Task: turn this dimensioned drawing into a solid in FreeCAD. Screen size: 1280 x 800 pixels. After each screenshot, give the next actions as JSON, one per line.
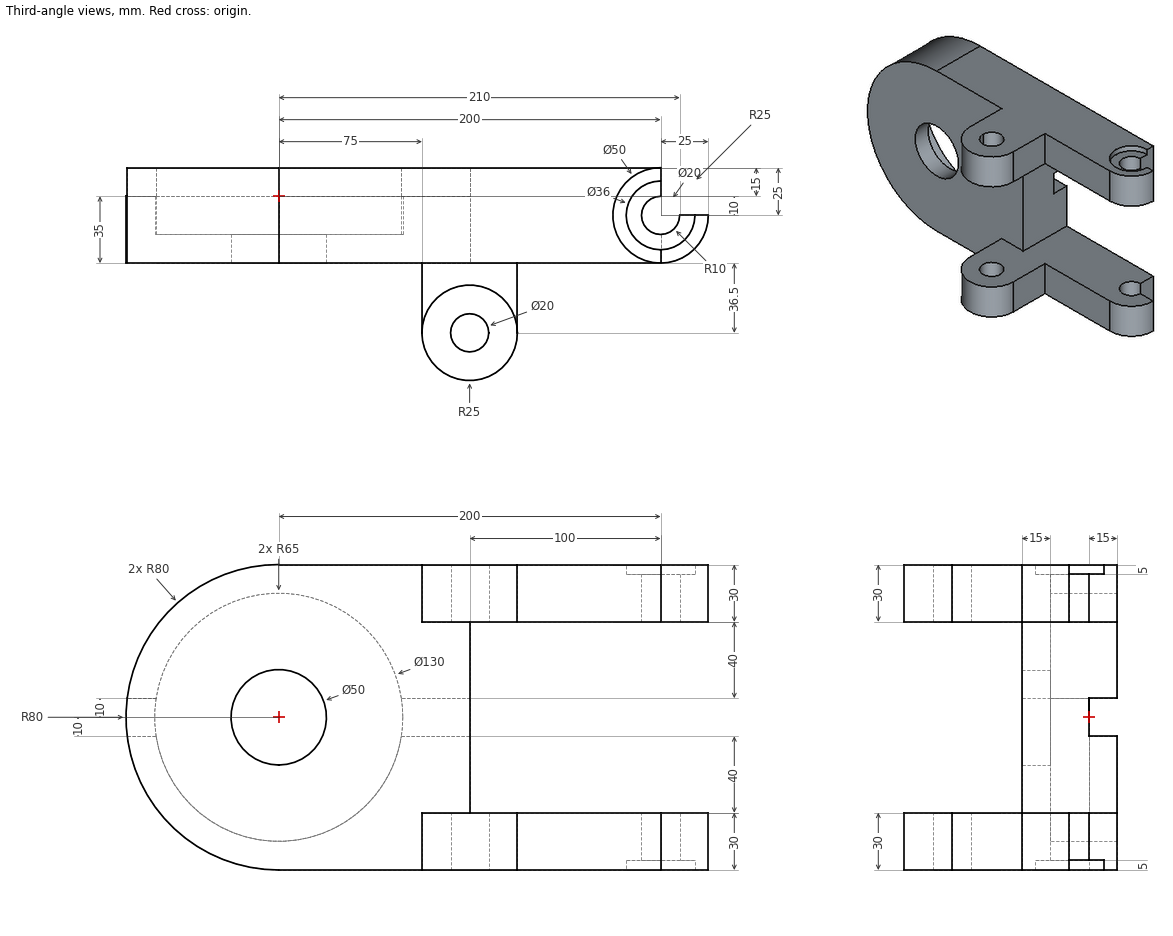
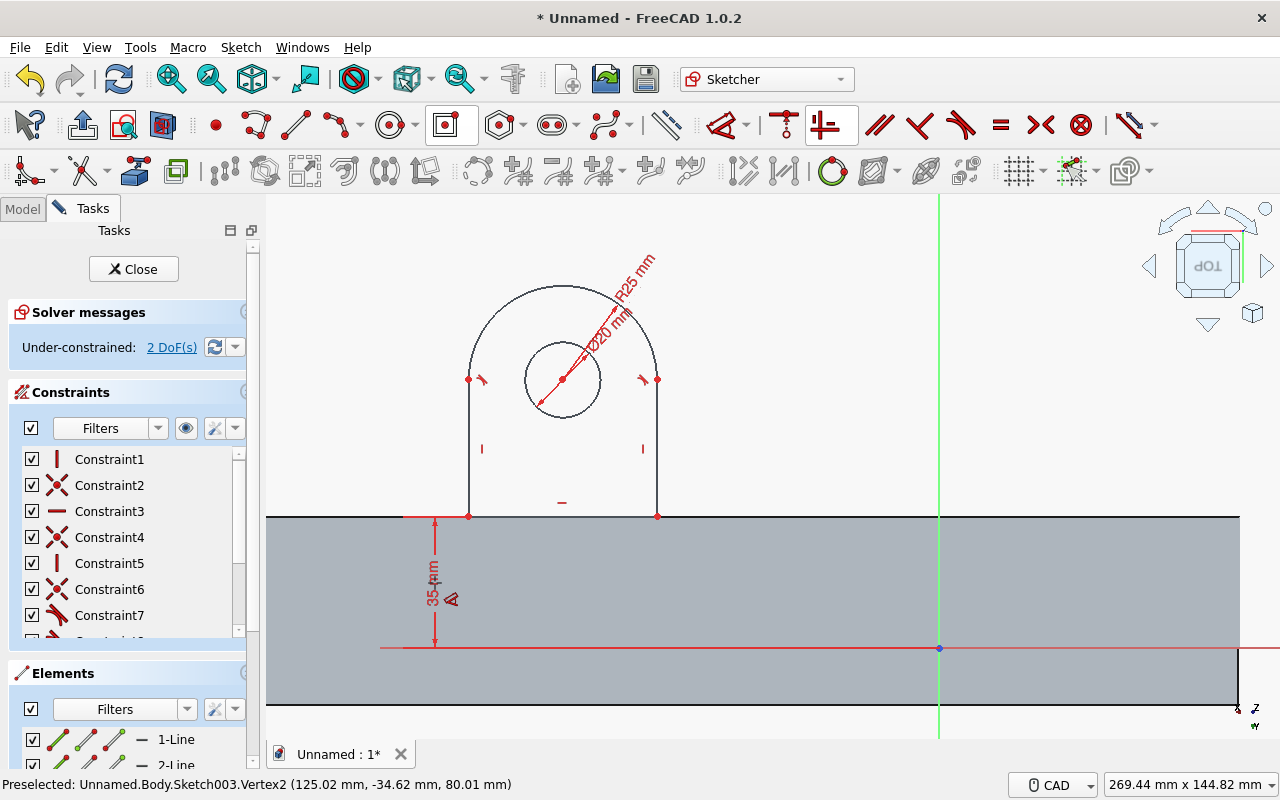
{"action": "left_click", "coordinate": [657, 517]}
{"action": "left_click", "coordinate": [798, 682]}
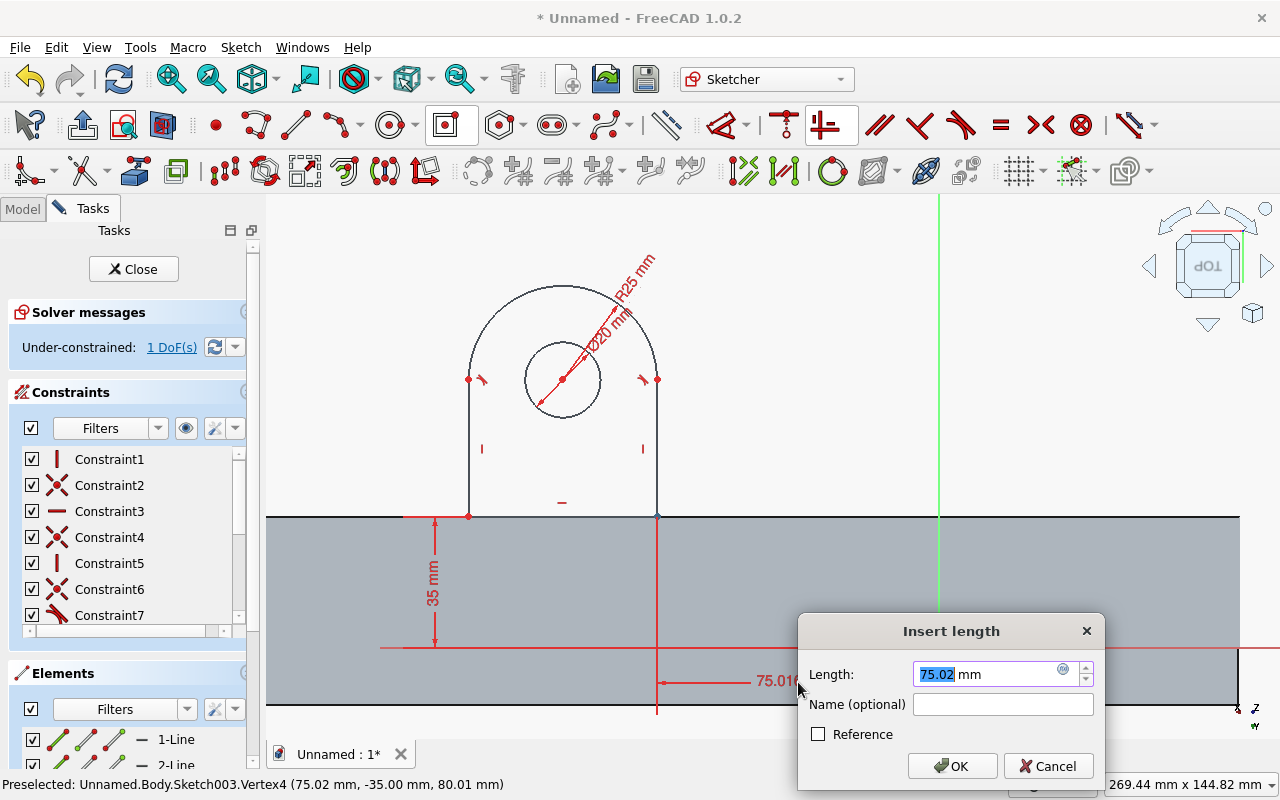
{"action": "type", "text": "75"}
{"action": "key", "text": "Return"}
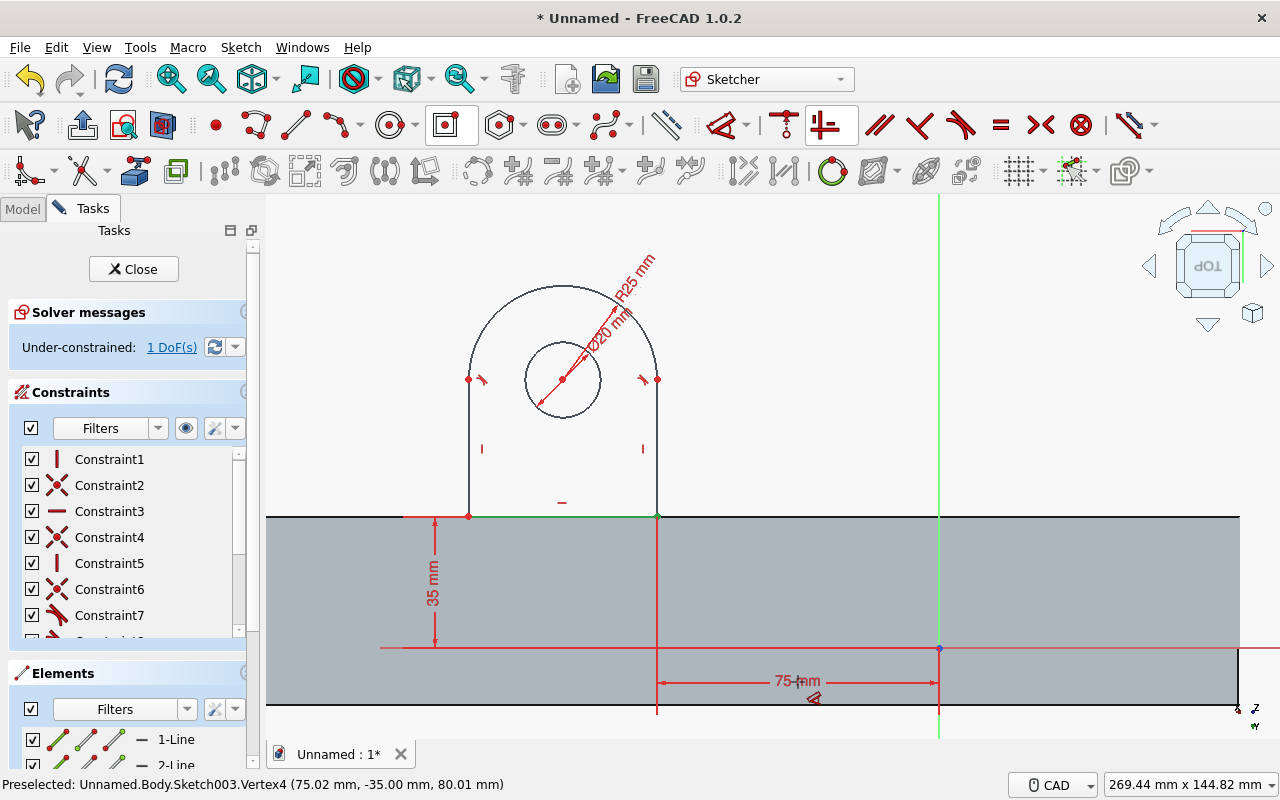
{"action": "left_click", "coordinate": [469, 421]}
{"action": "left_click", "coordinate": [435, 448]}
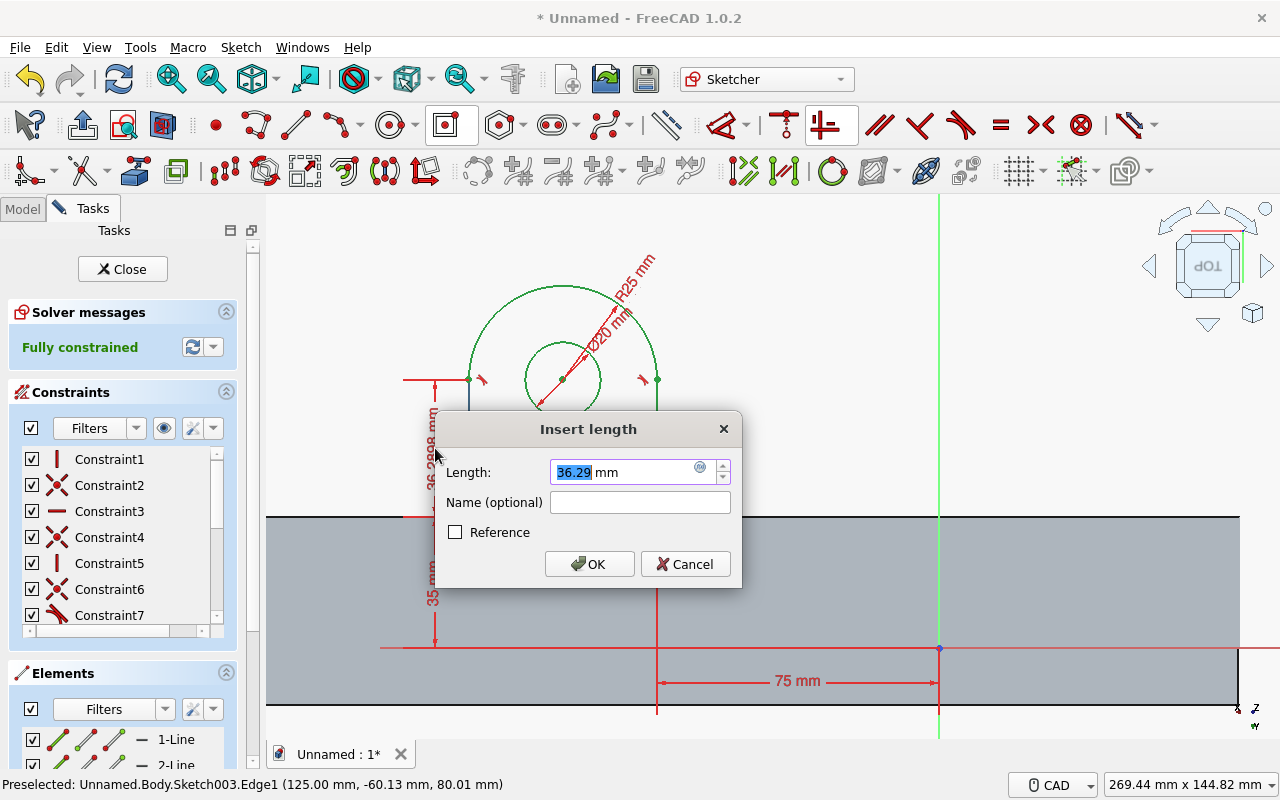
{"action": "type", "text": "36.5"}
{"action": "key", "text": "Return"}
{"action": "key", "text": "Escape"}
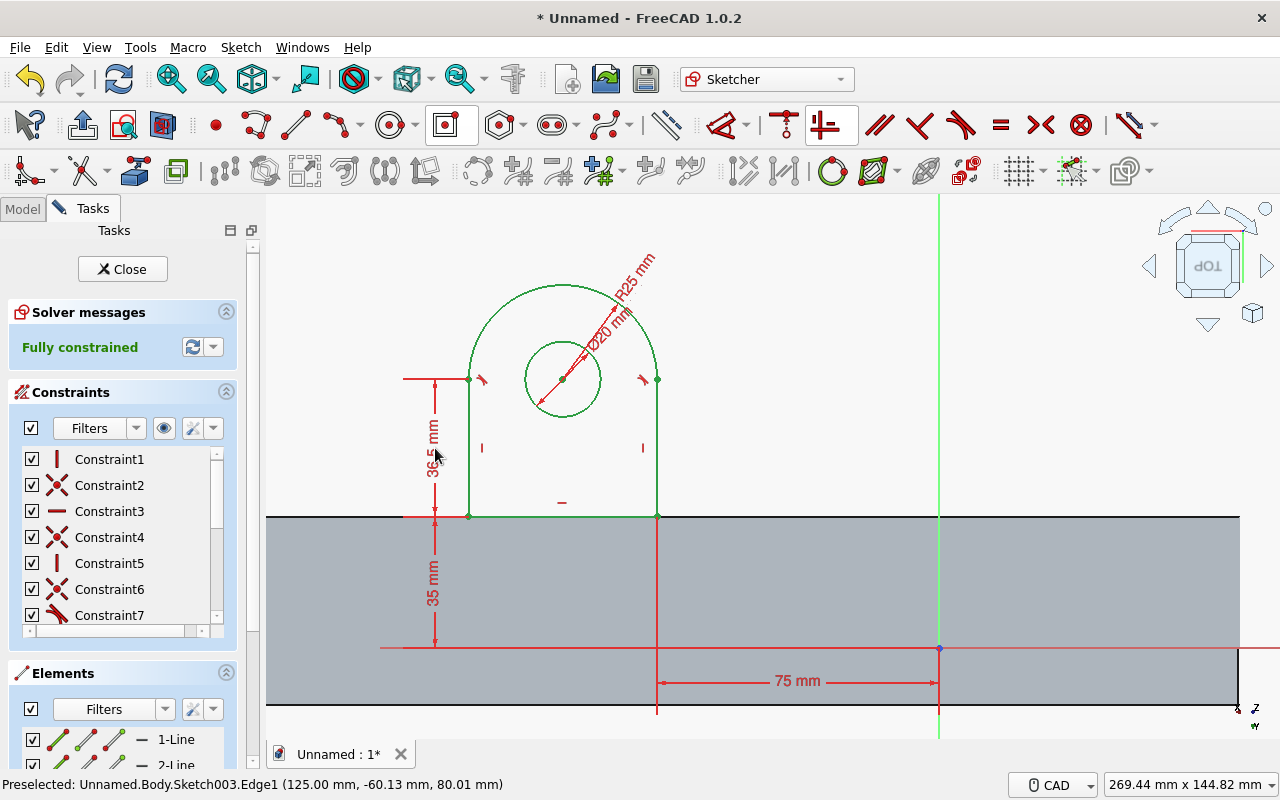
{"action": "left_click", "coordinate": [123, 269]}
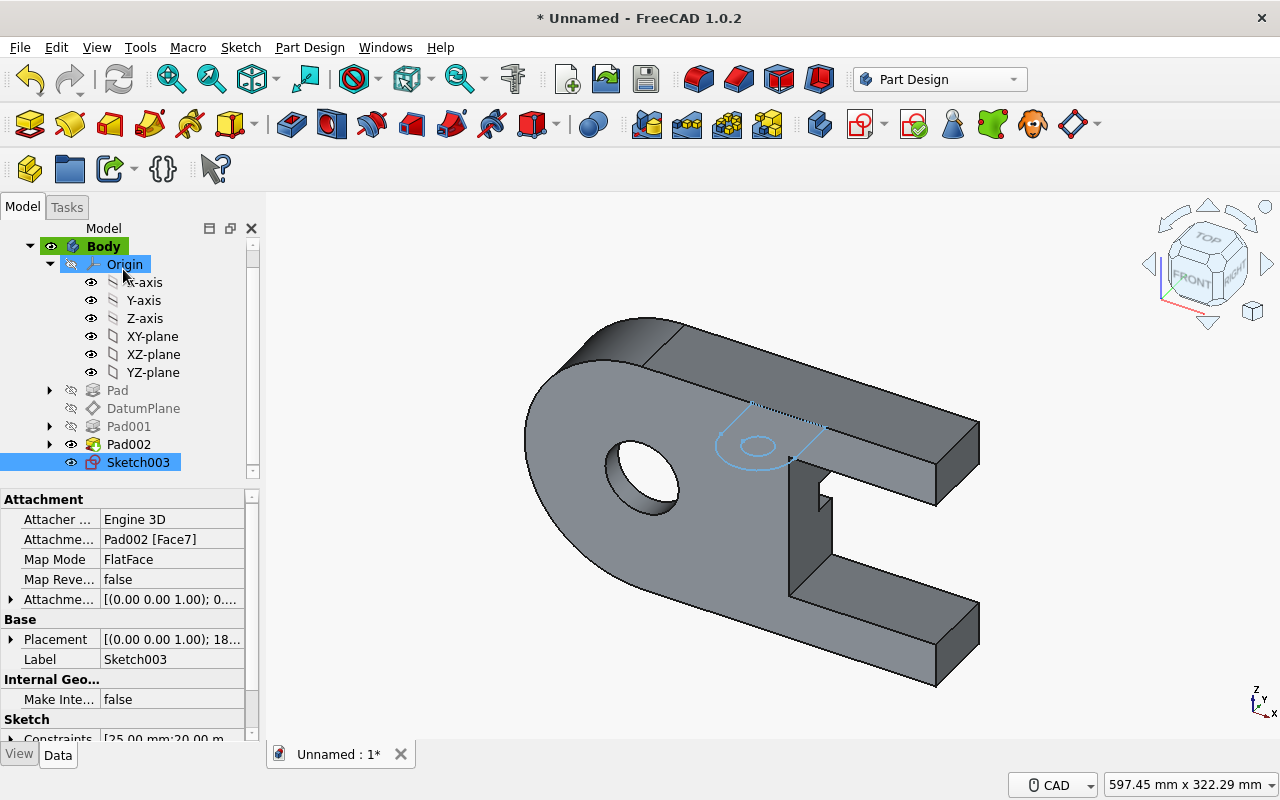
{"action": "left_click", "coordinate": [30, 124]}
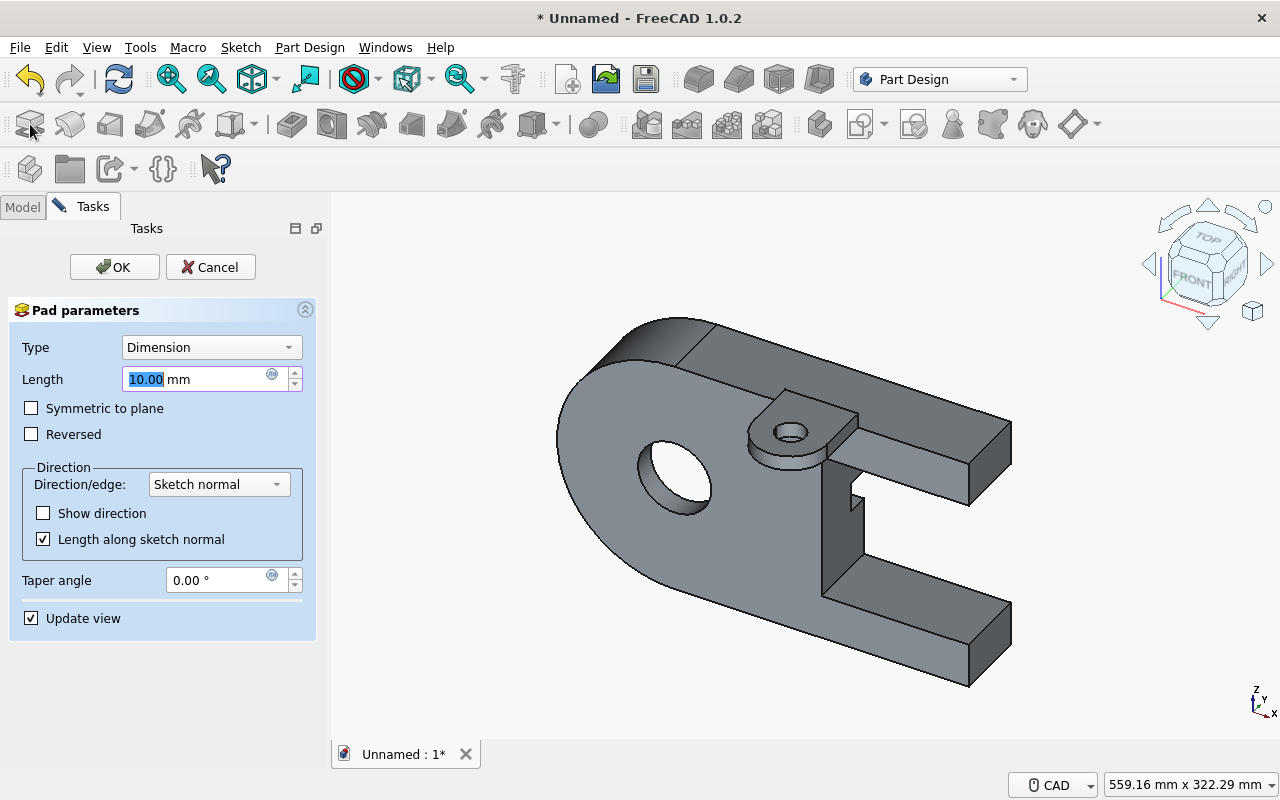
{"action": "type", "text": "30"}
{"action": "key", "text": "Tab"}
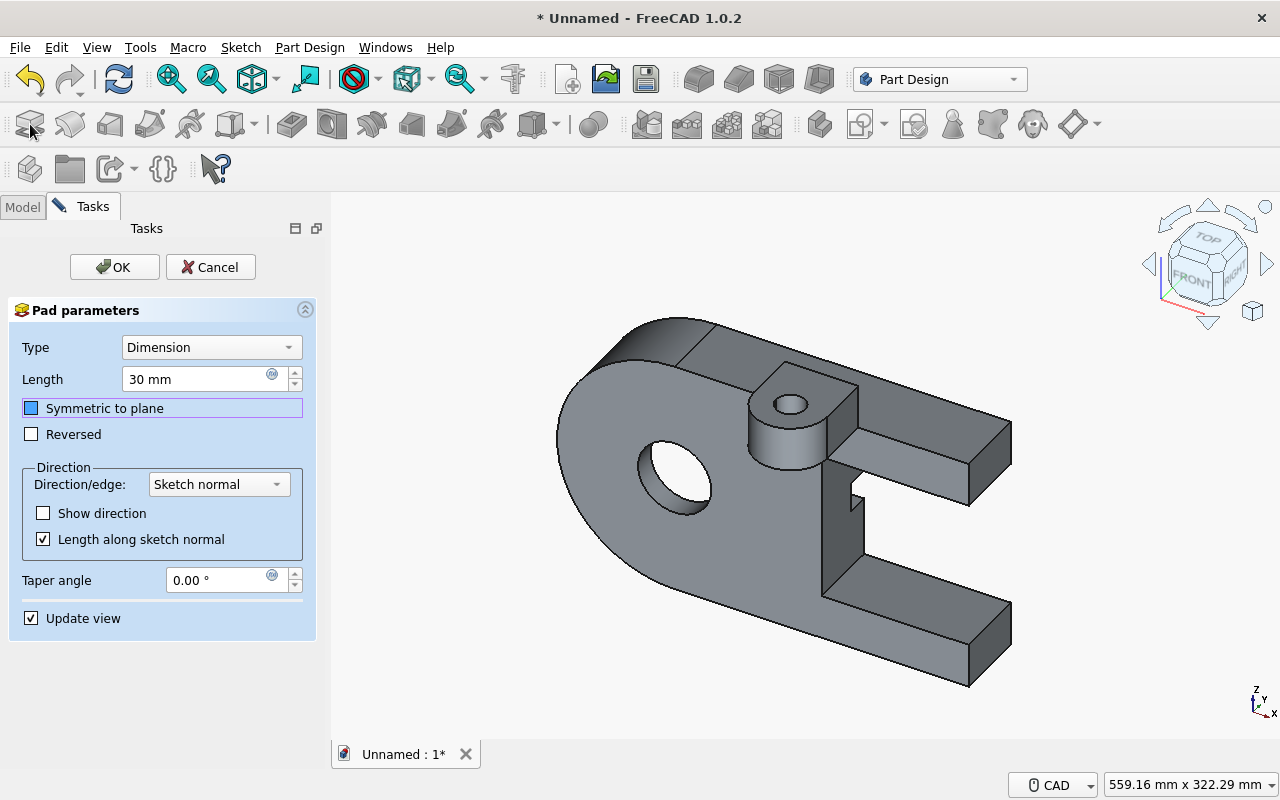
{"action": "left_click", "coordinate": [30, 434]}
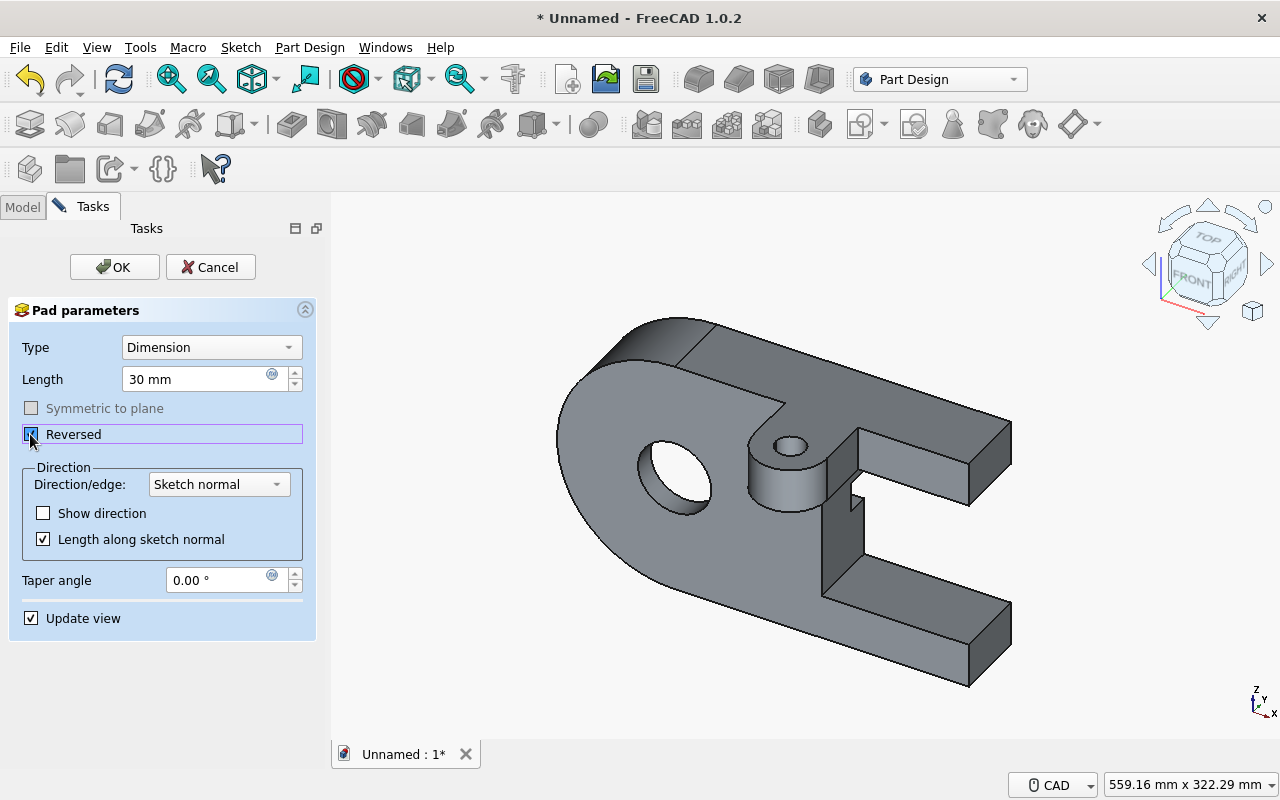
{"action": "left_click", "coordinate": [115, 267]}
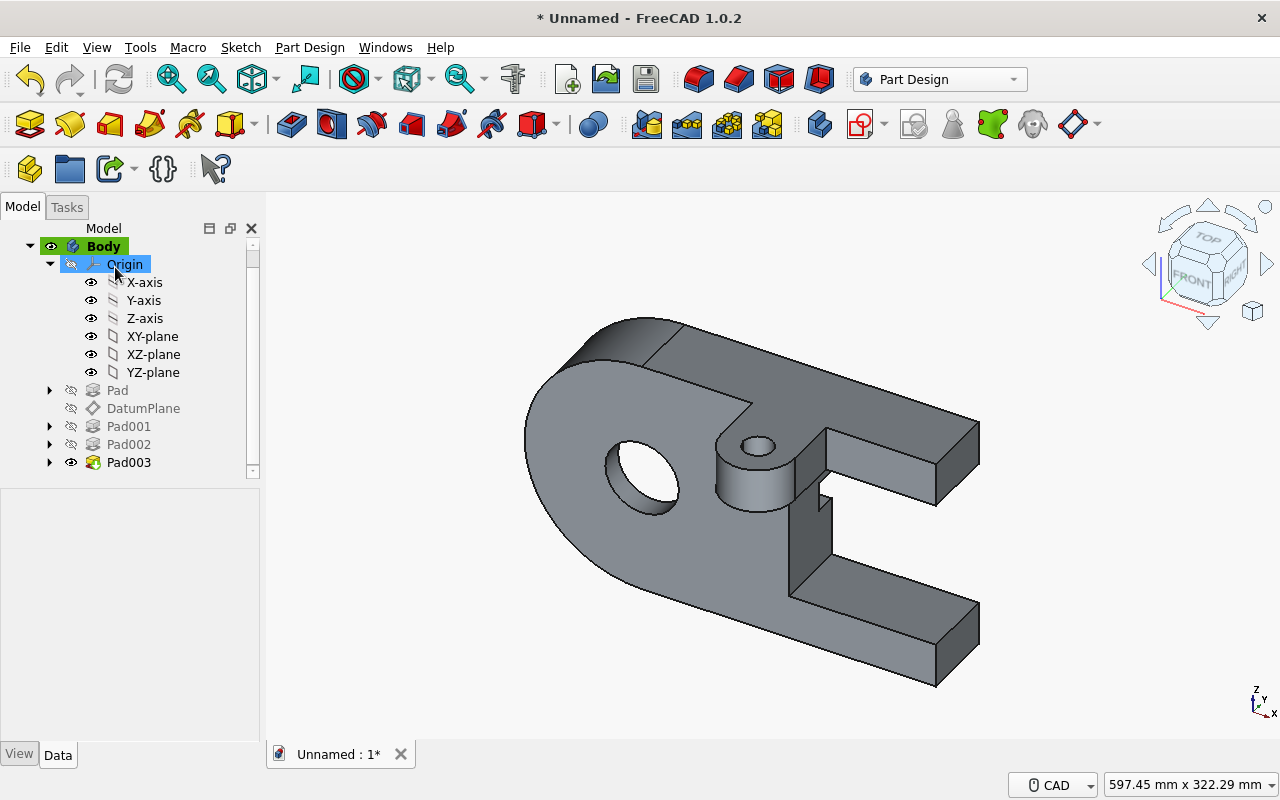
{"action": "left_click", "coordinate": [136, 336]}